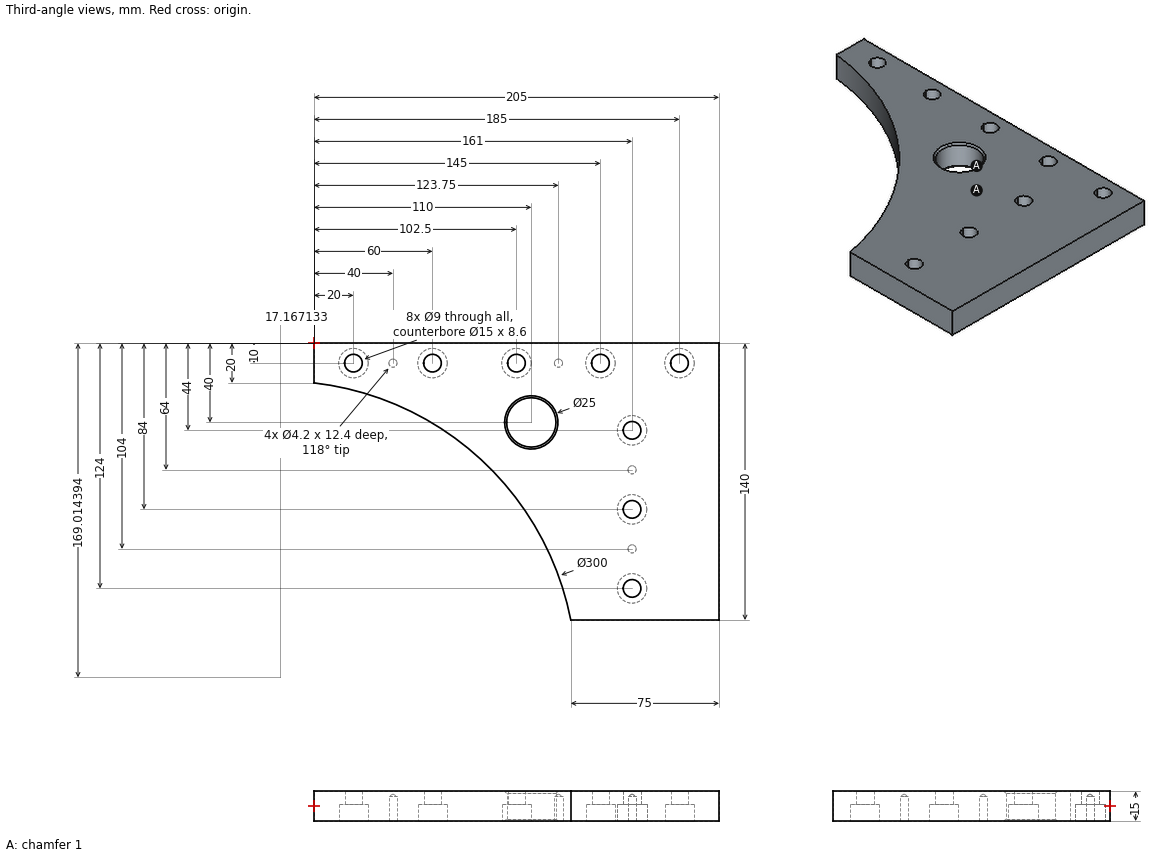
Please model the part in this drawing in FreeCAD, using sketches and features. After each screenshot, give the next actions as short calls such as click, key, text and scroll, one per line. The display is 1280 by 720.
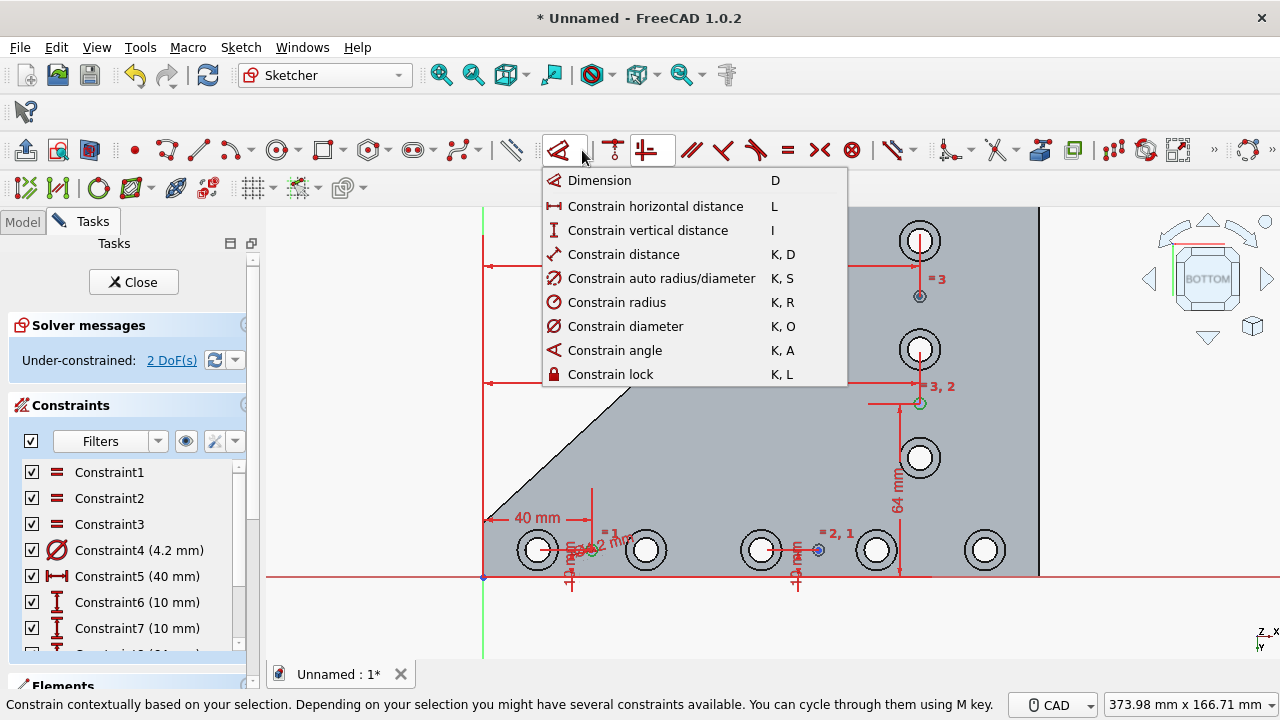
click(695, 230)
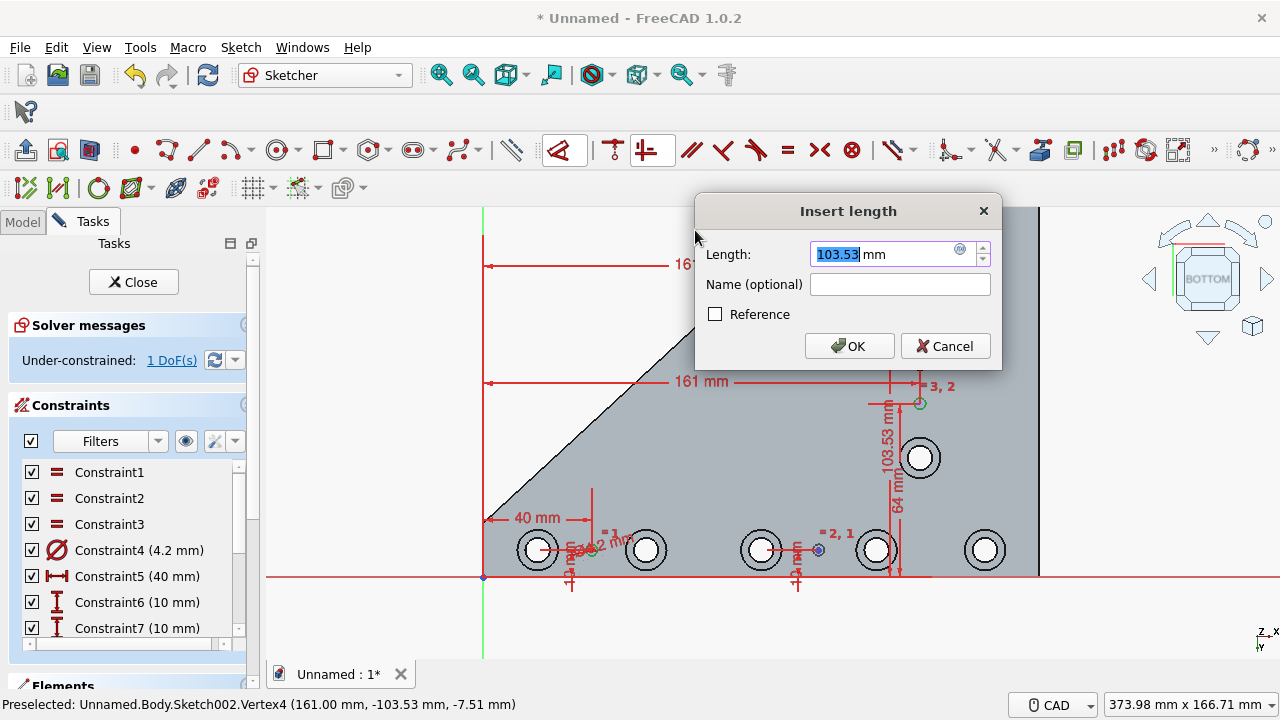
text(104)
key(Return)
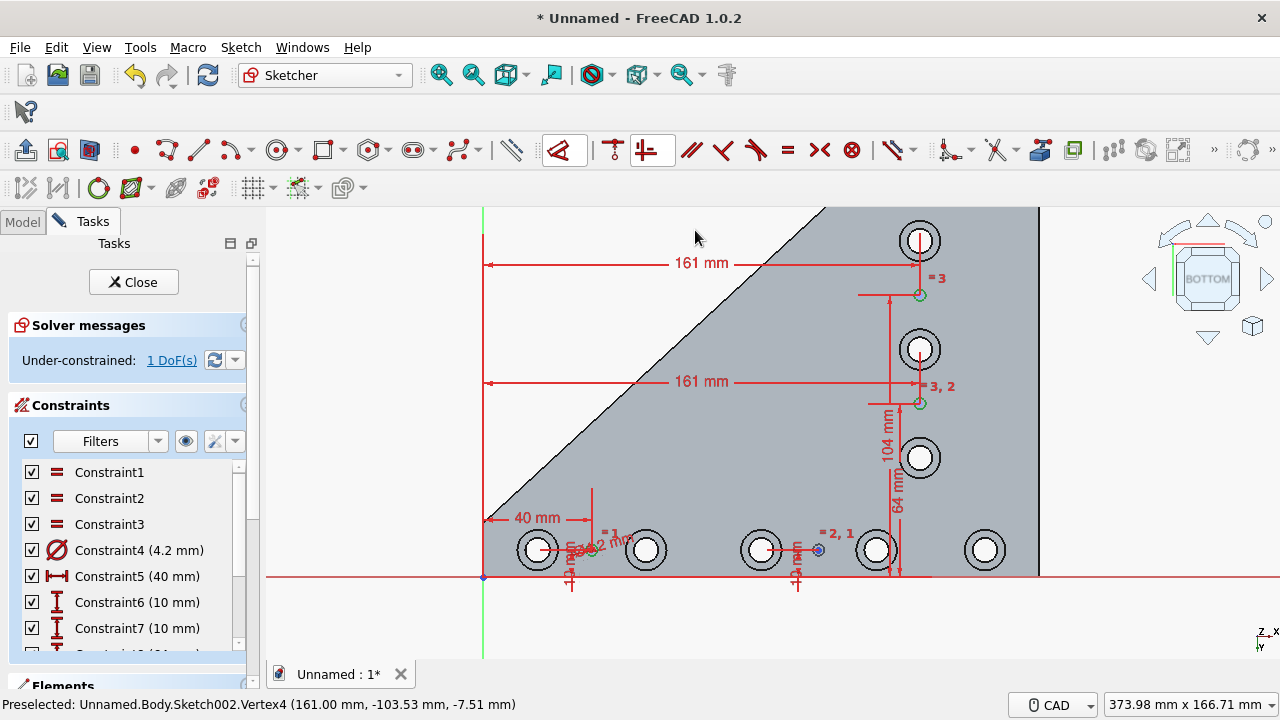
click(819, 550)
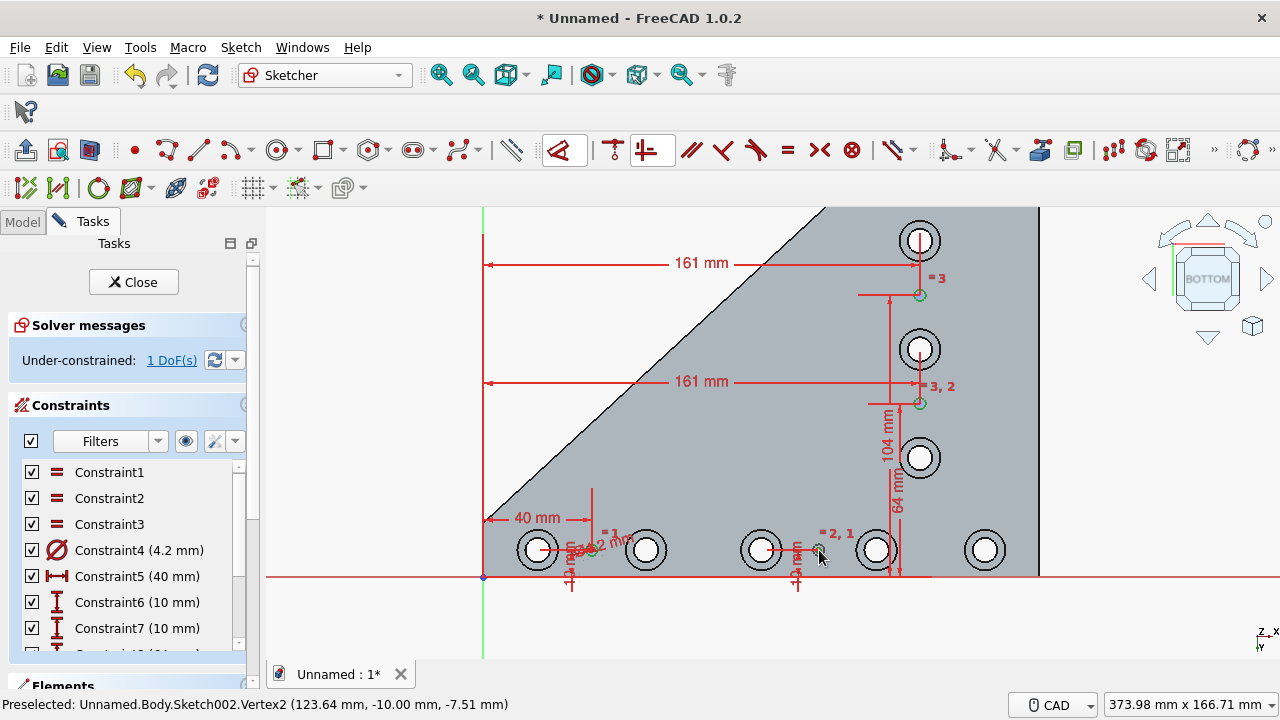
key(l)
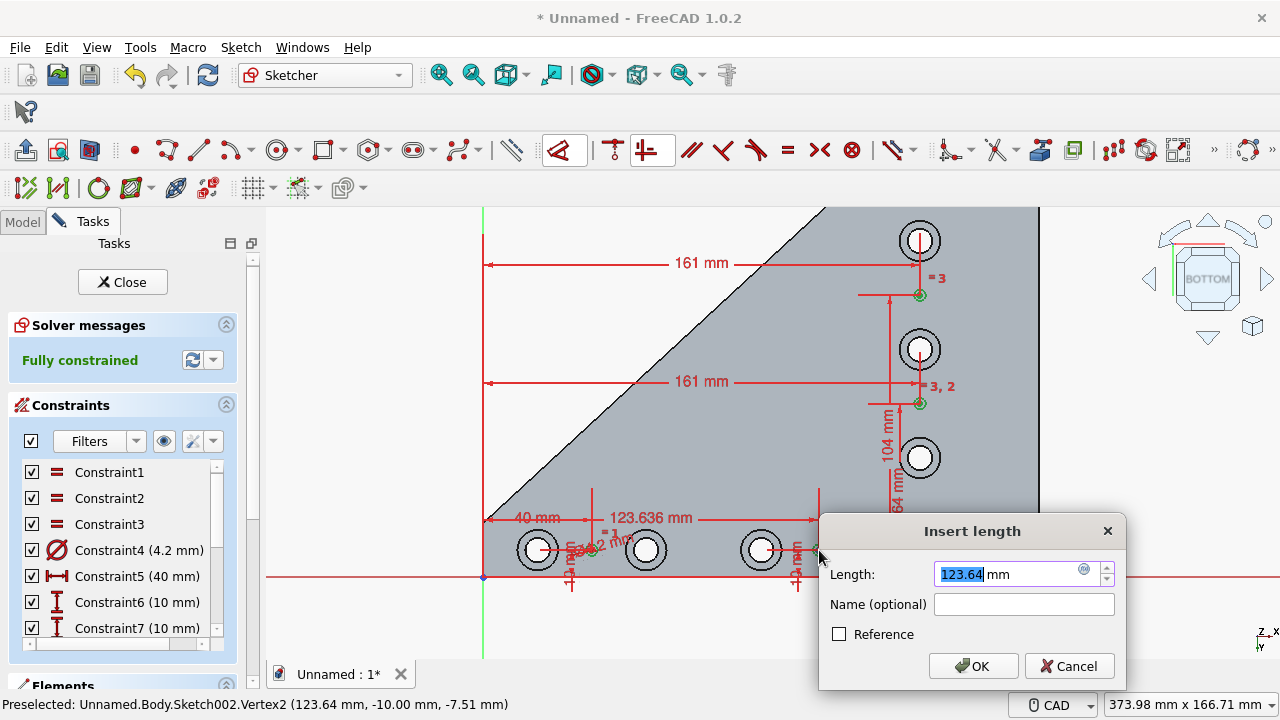
text(123.75)
key(Return)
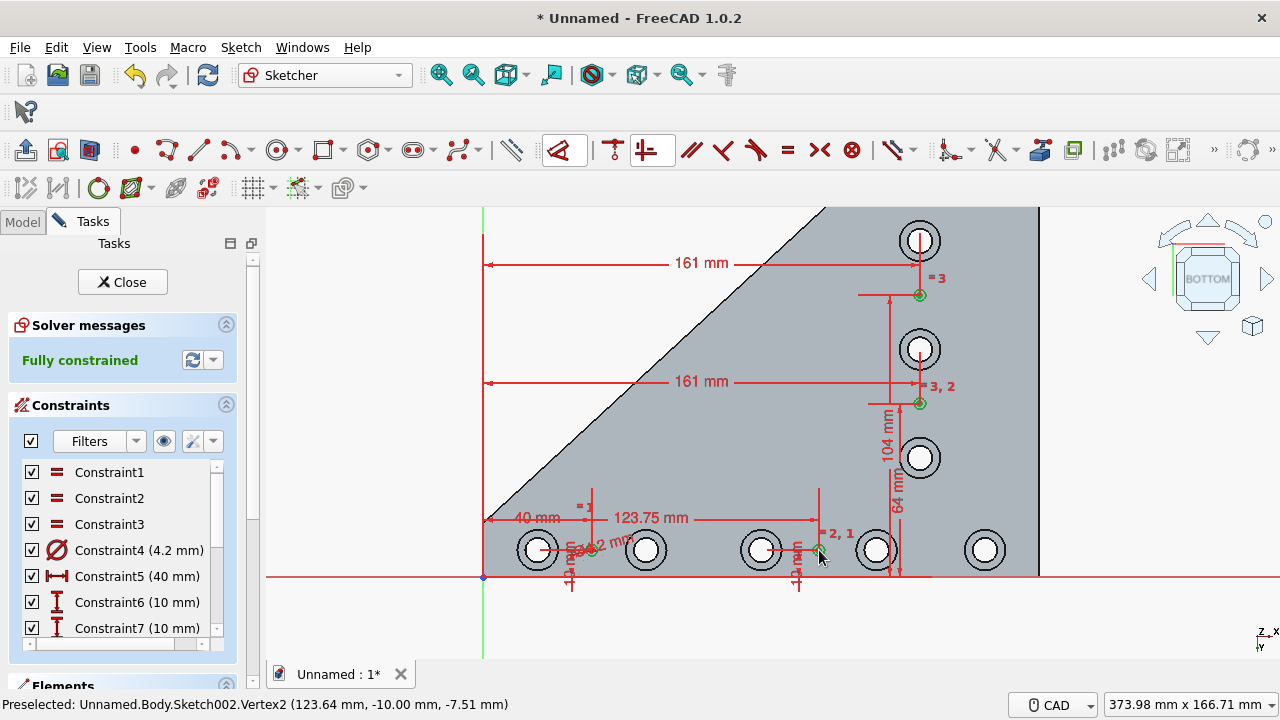
click(123, 282)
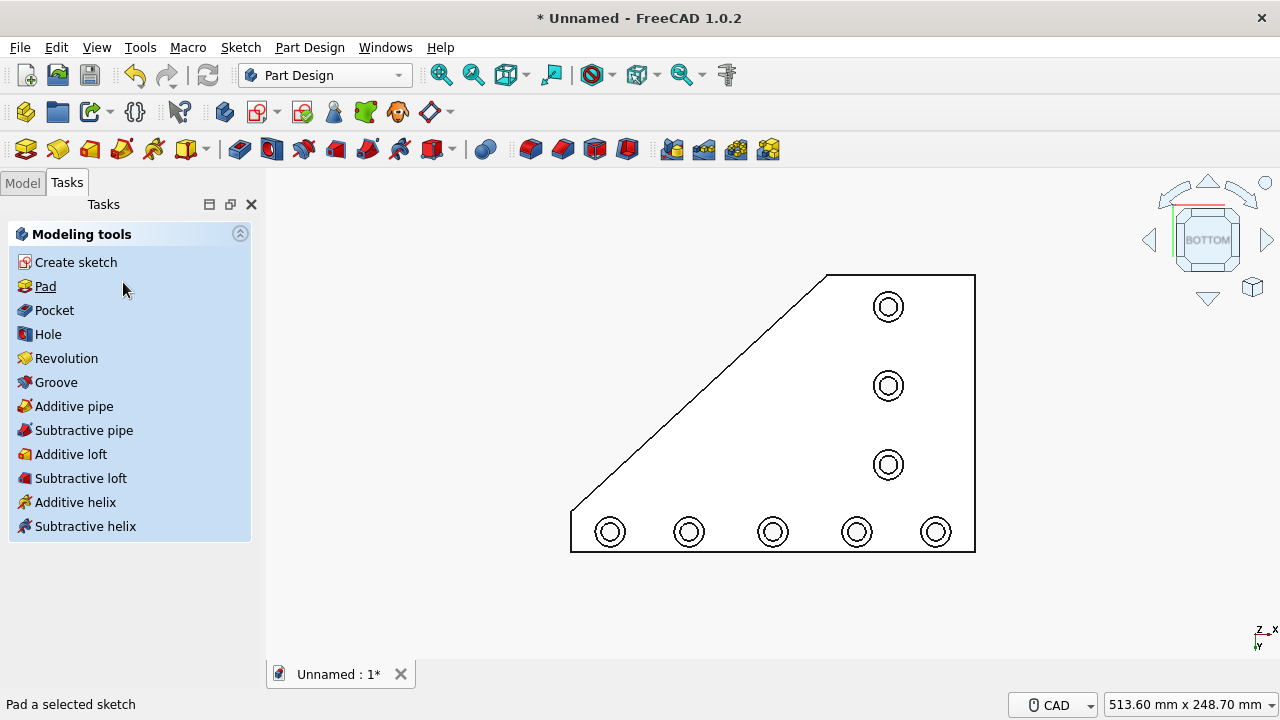
click(272, 150)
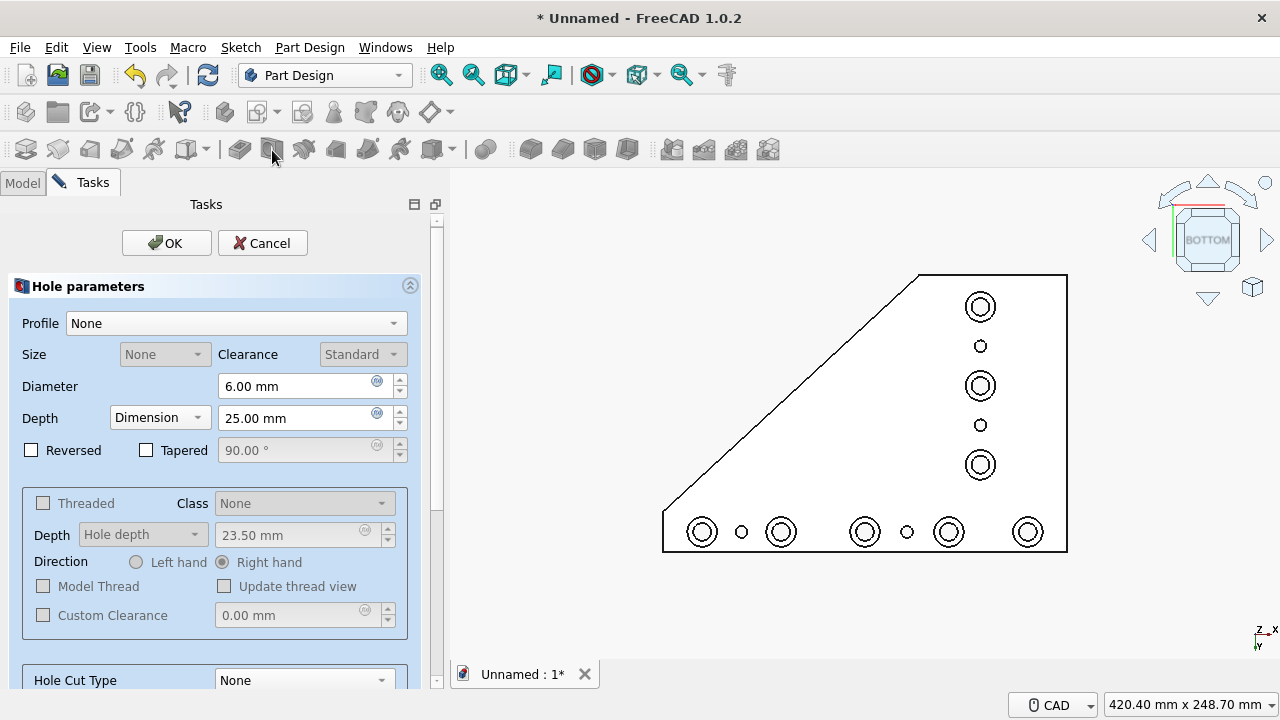
triple_click(305, 386)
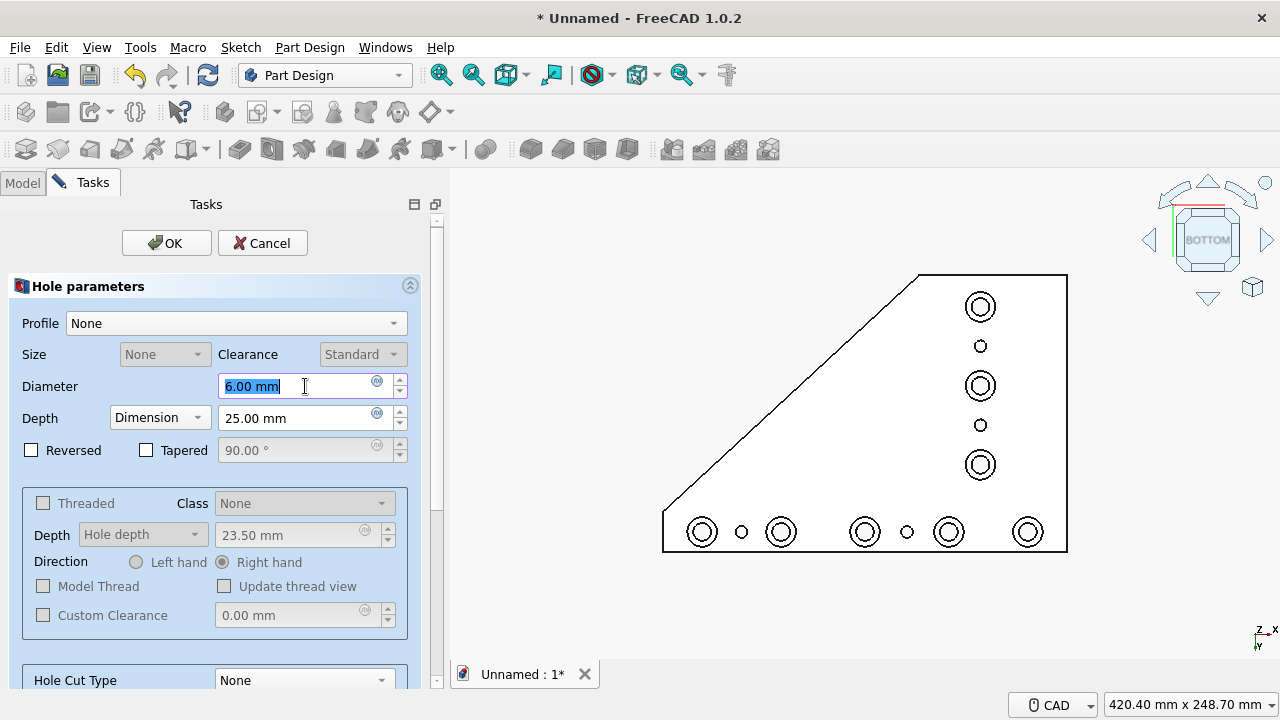
text(4.2)
key(Tab)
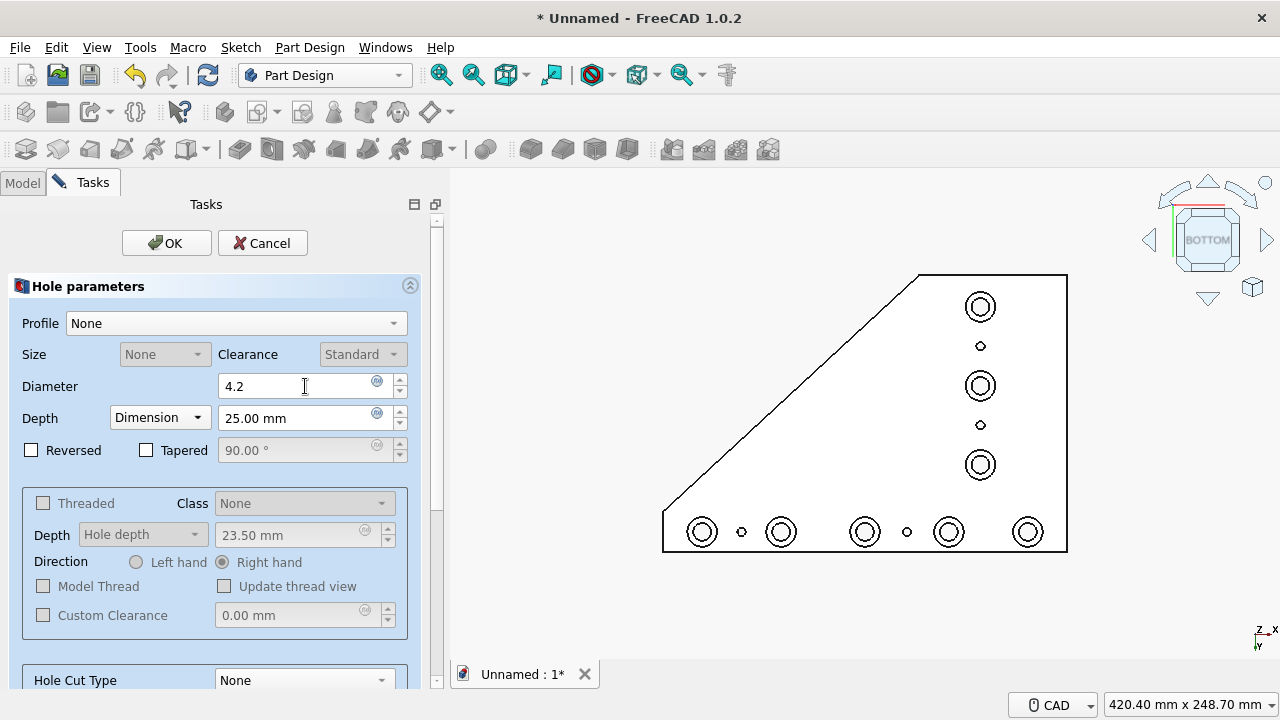
triple_click(305, 418)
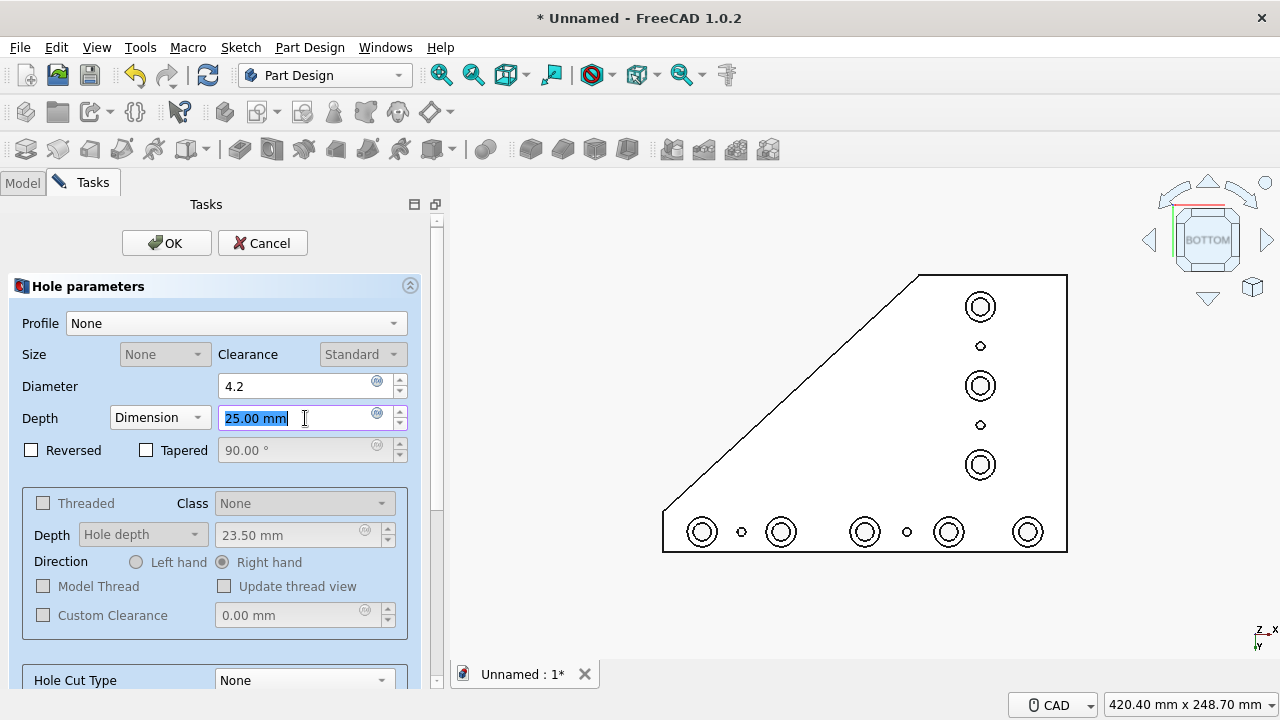
text(12.4)
key(Tab)